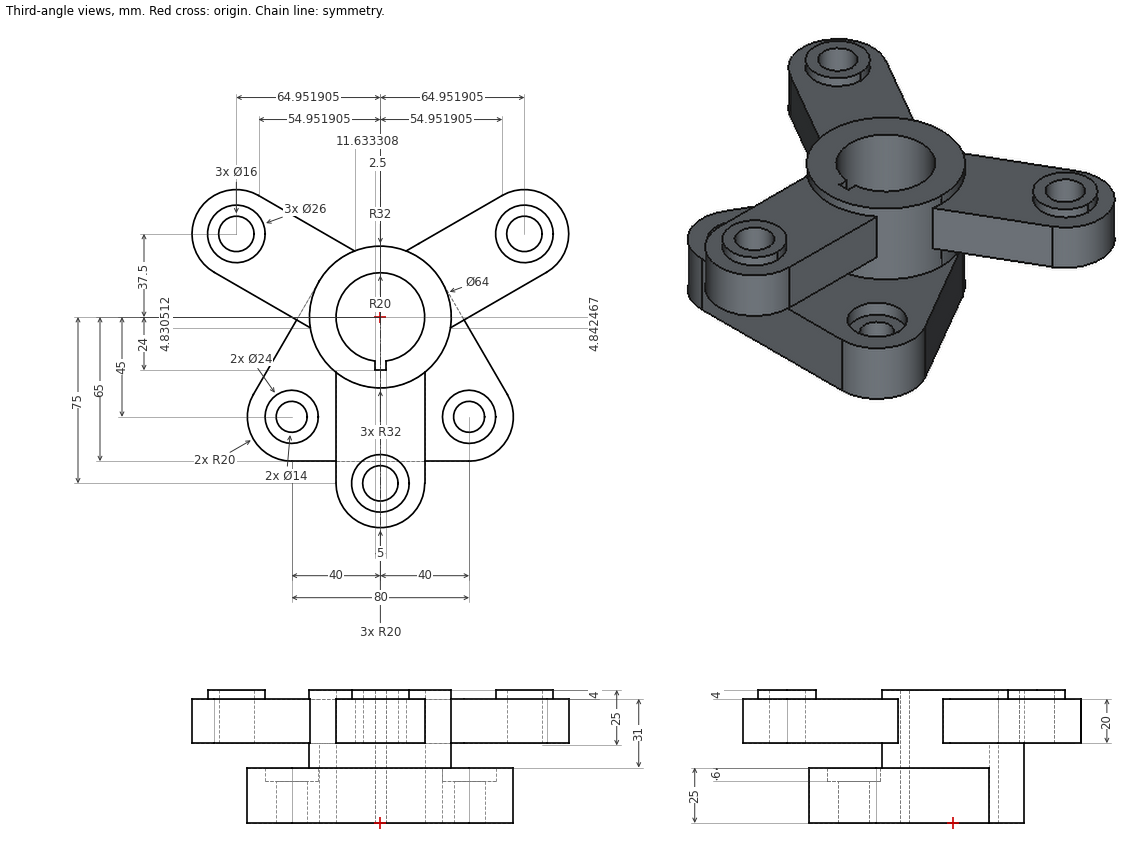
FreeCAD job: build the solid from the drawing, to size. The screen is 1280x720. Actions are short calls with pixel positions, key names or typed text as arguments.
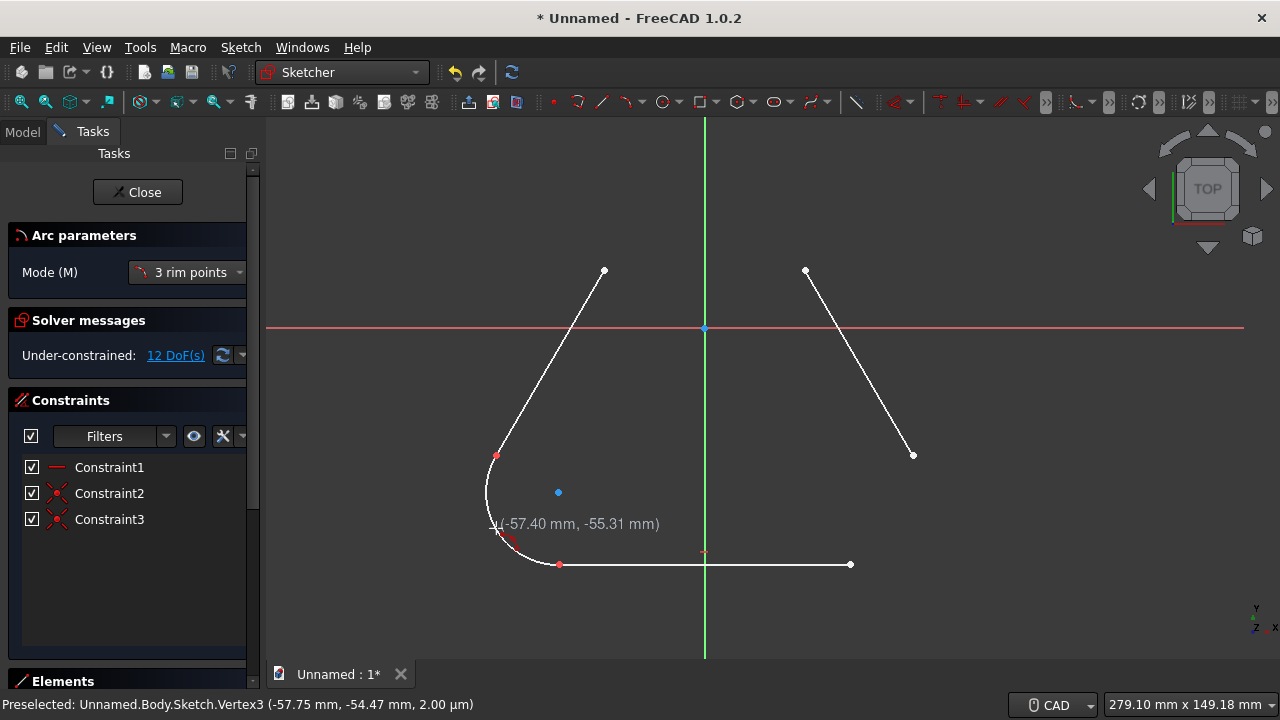
click(850, 565)
click(913, 456)
click(913, 528)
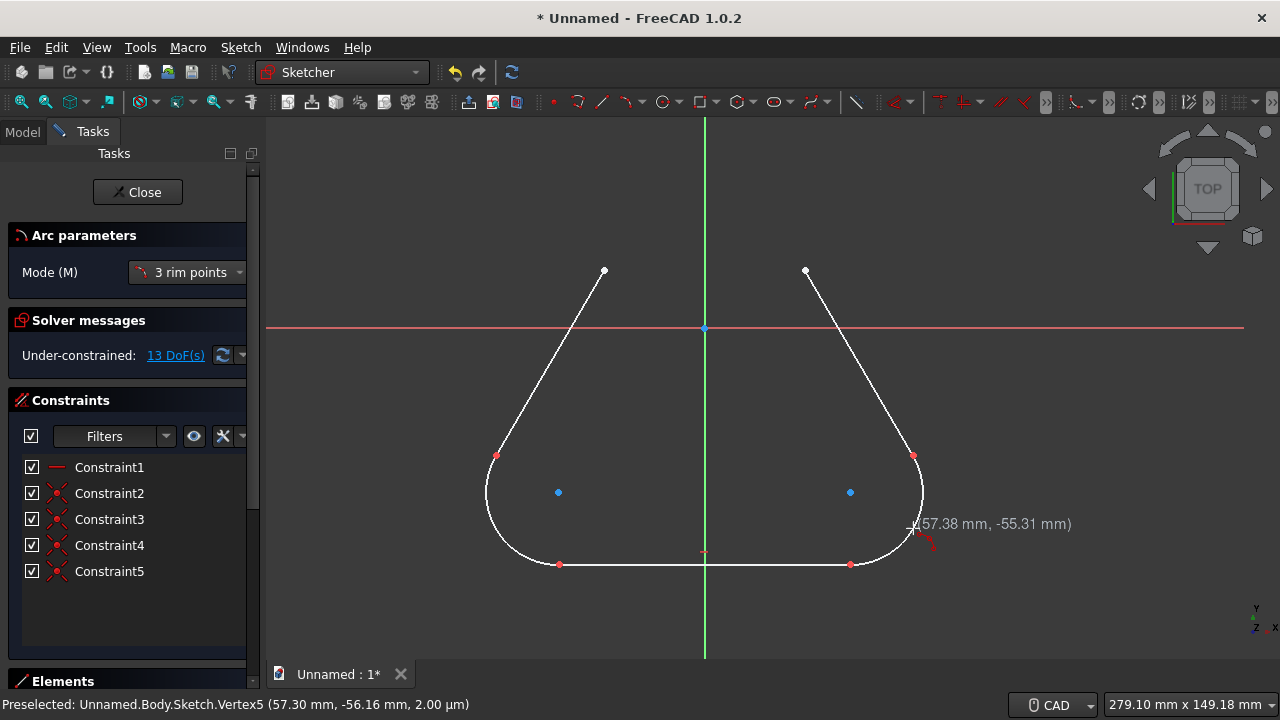
click(805, 271)
click(604, 271)
click(729, 214)
key(Escape)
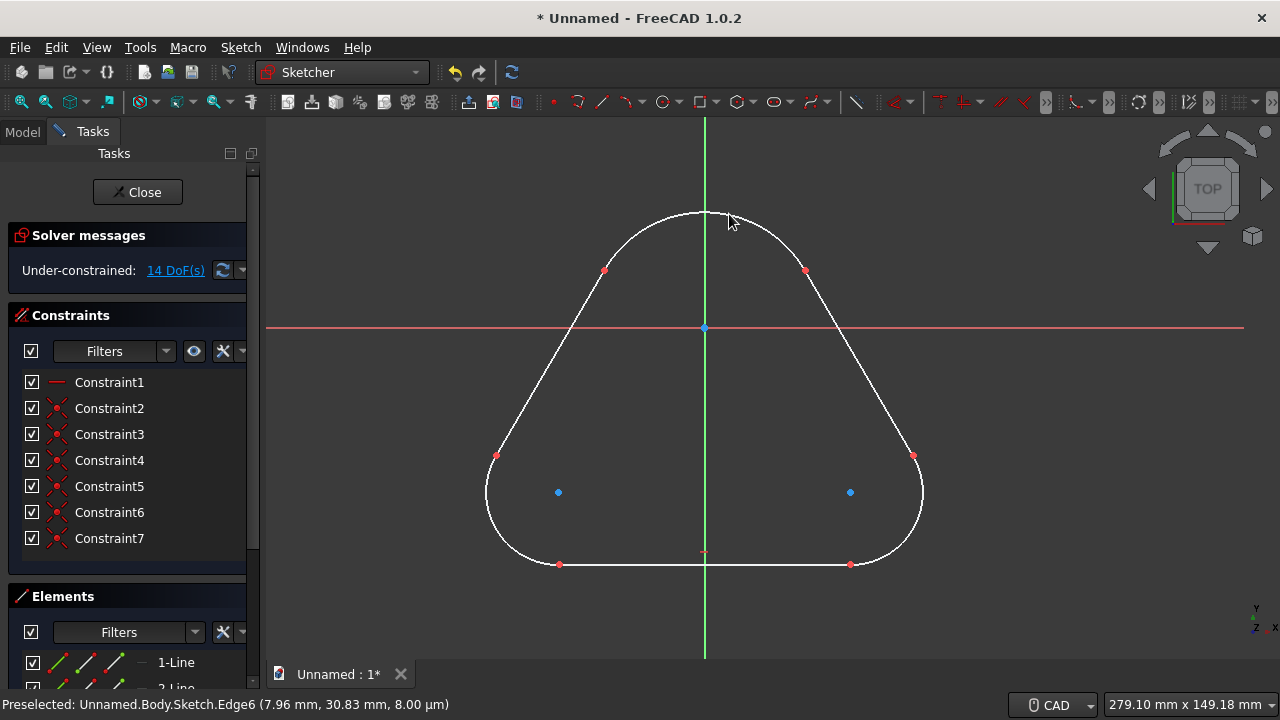
click(572, 327)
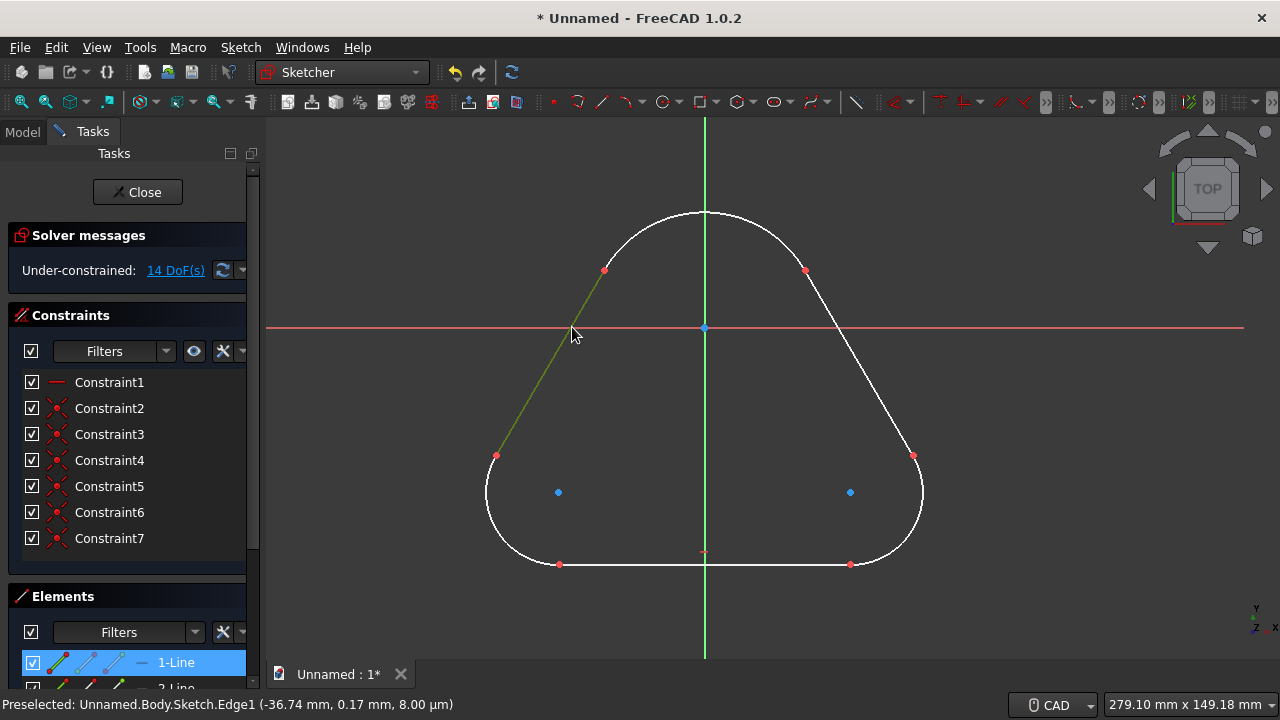
click(487, 500)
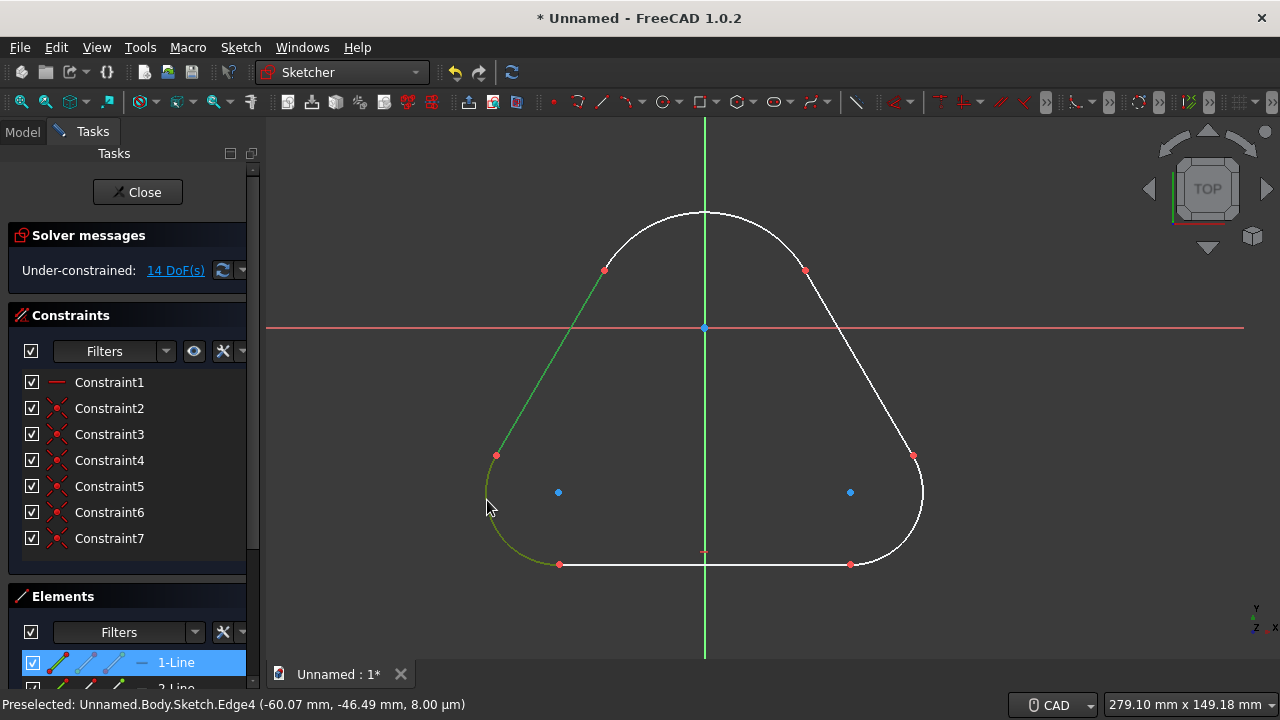
key(t)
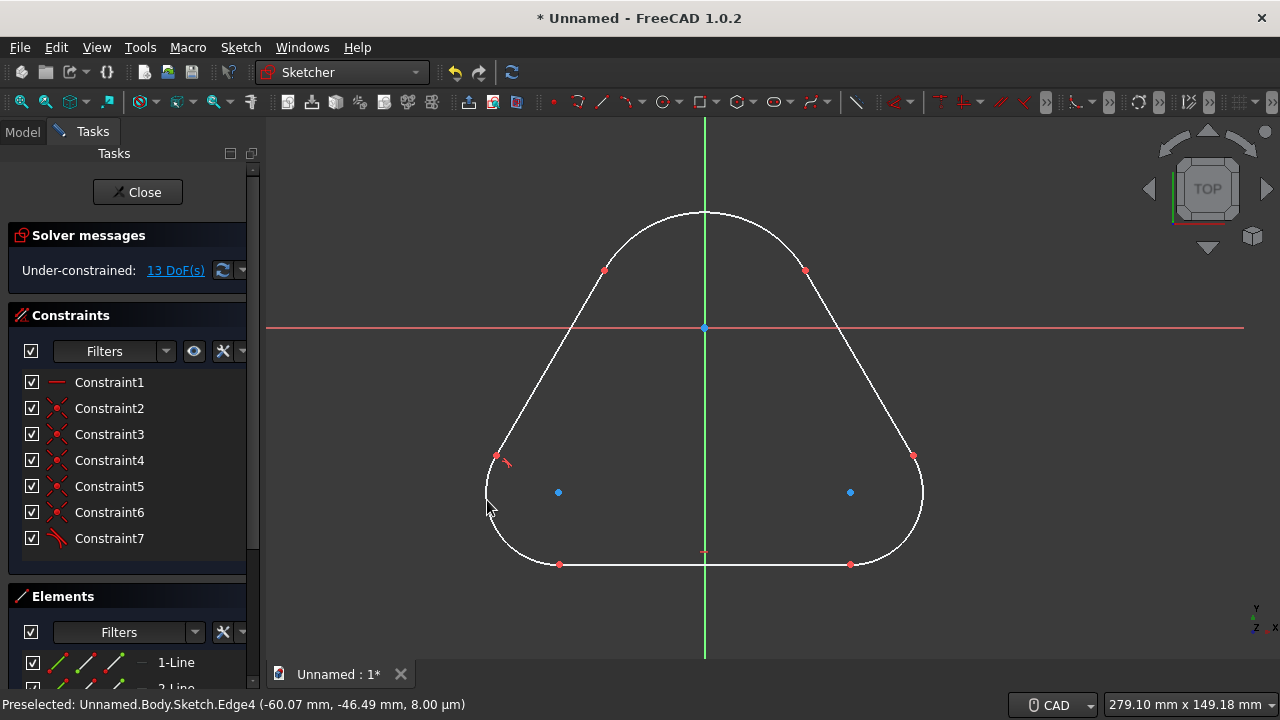
click(572, 327)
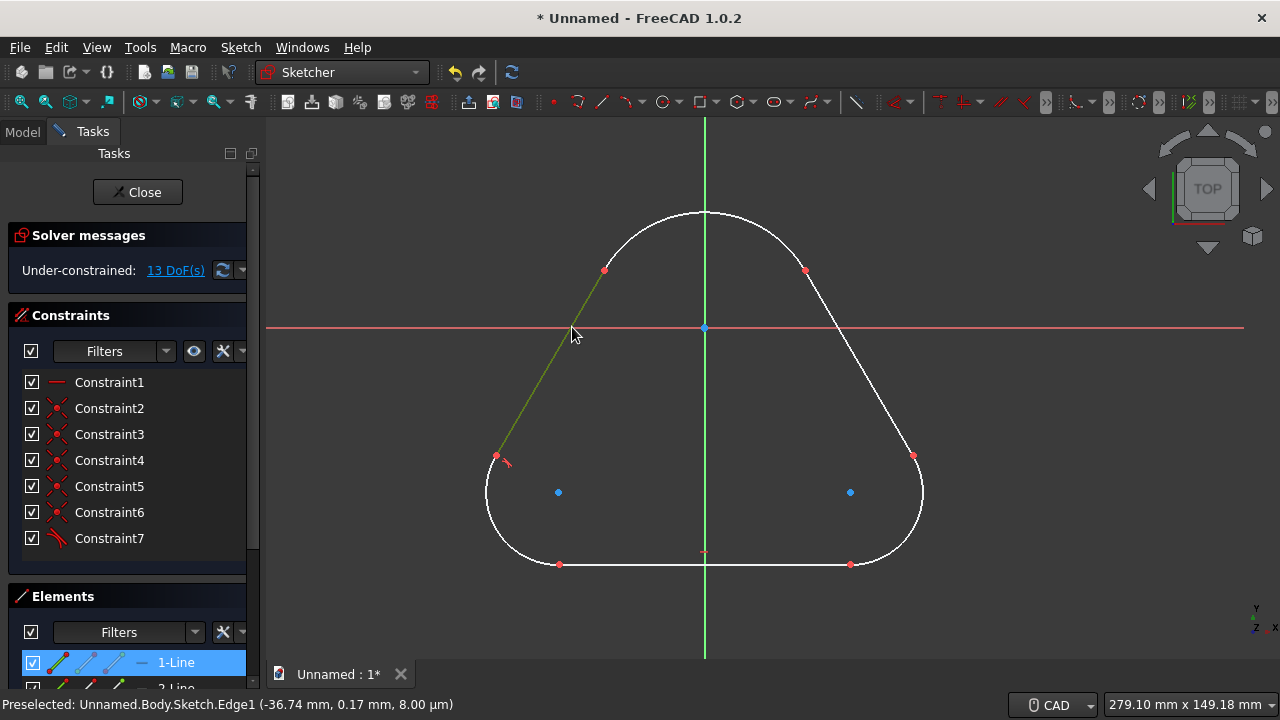
click(752, 223)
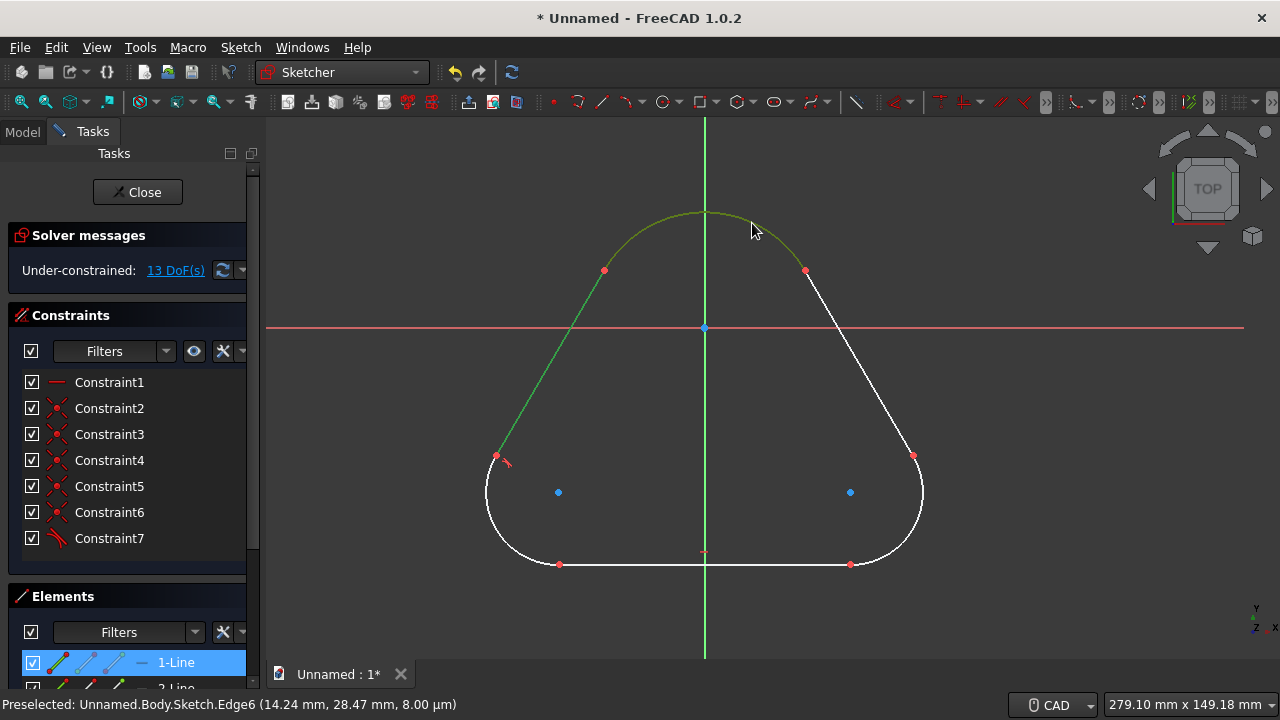
key(t)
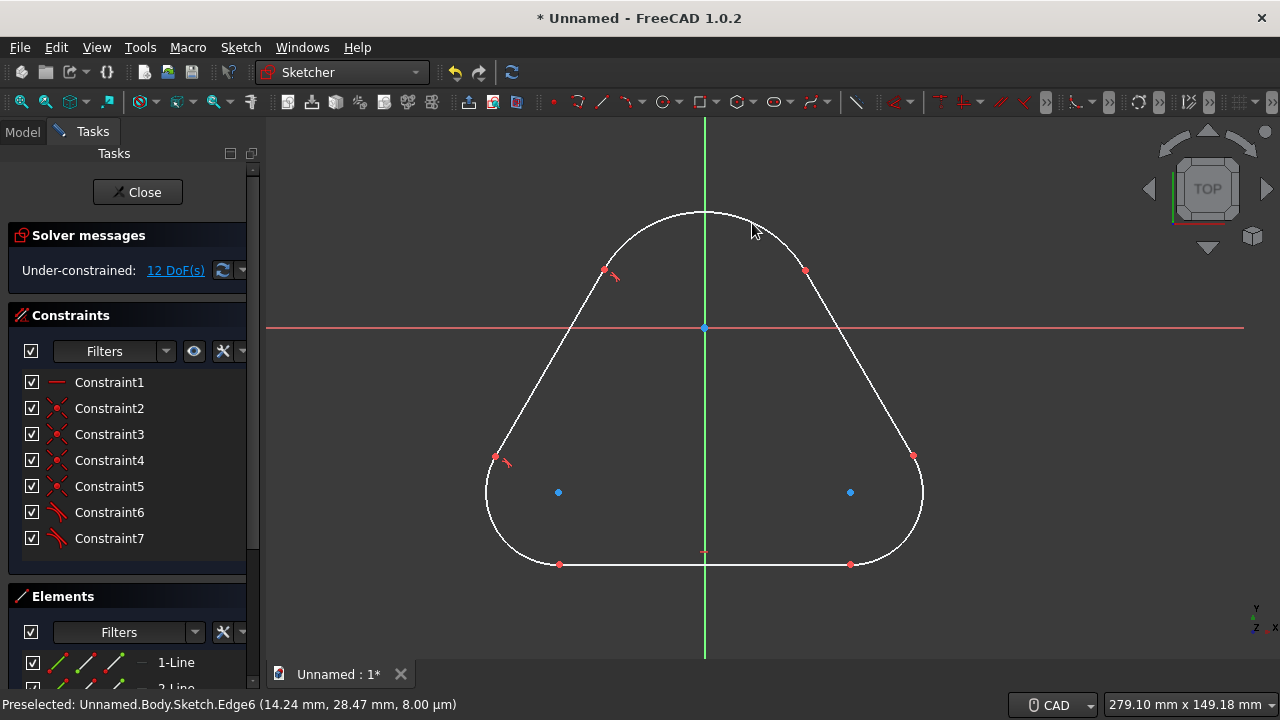
click(646, 565)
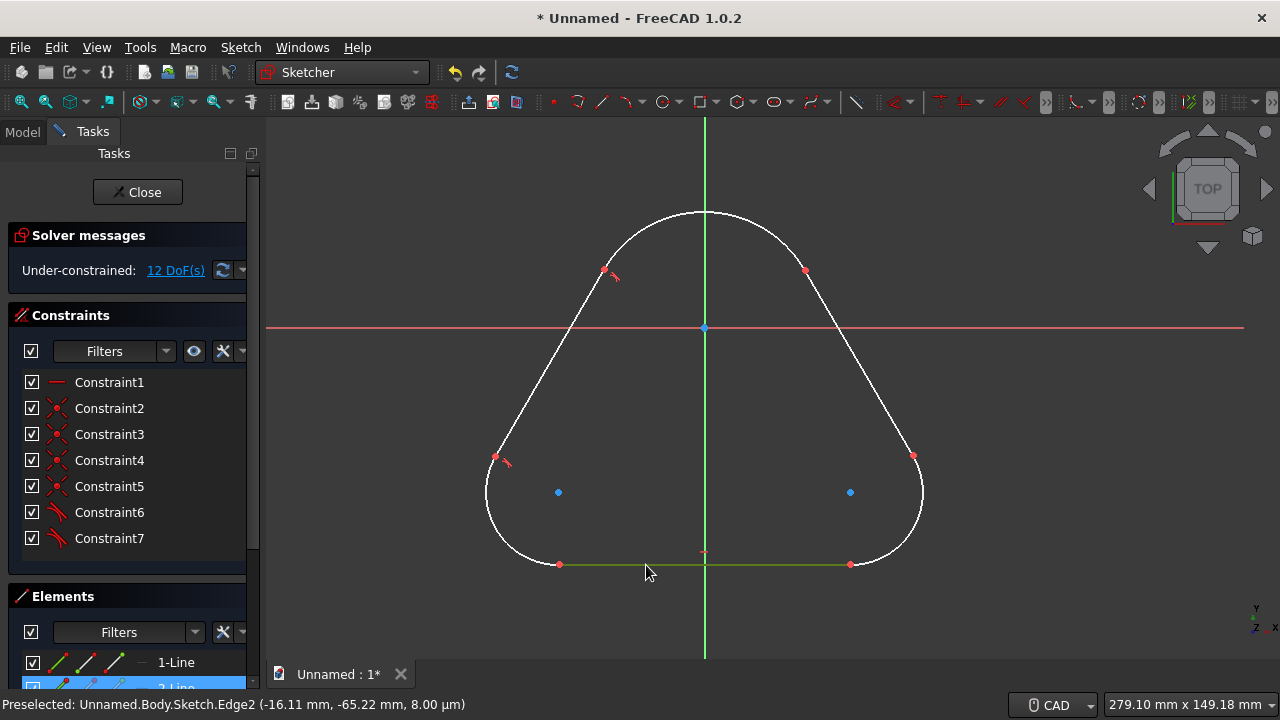
click(486, 500)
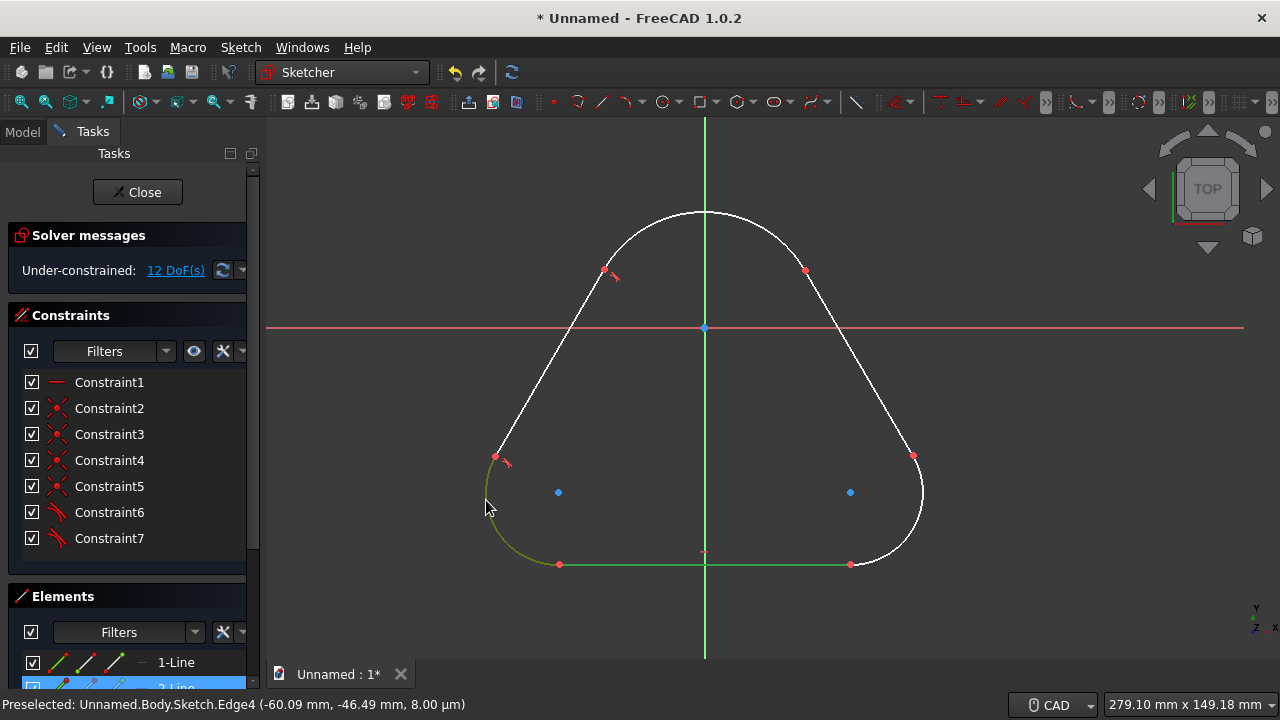
key(t)